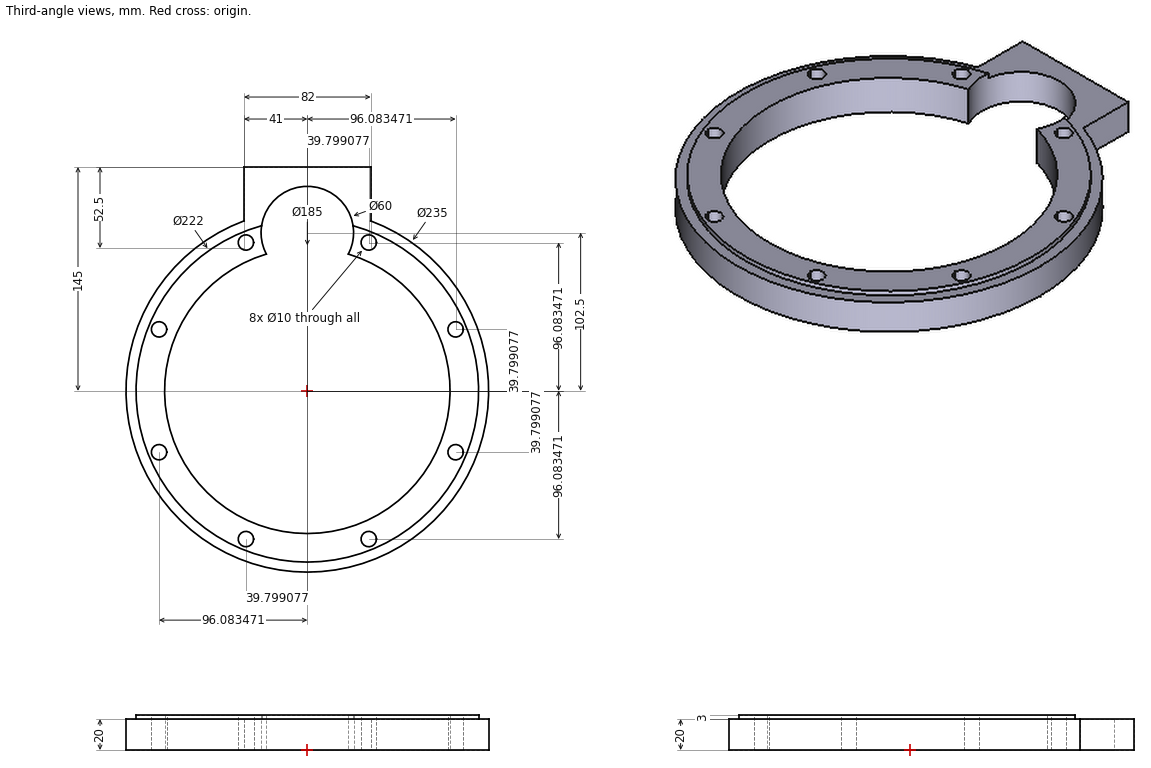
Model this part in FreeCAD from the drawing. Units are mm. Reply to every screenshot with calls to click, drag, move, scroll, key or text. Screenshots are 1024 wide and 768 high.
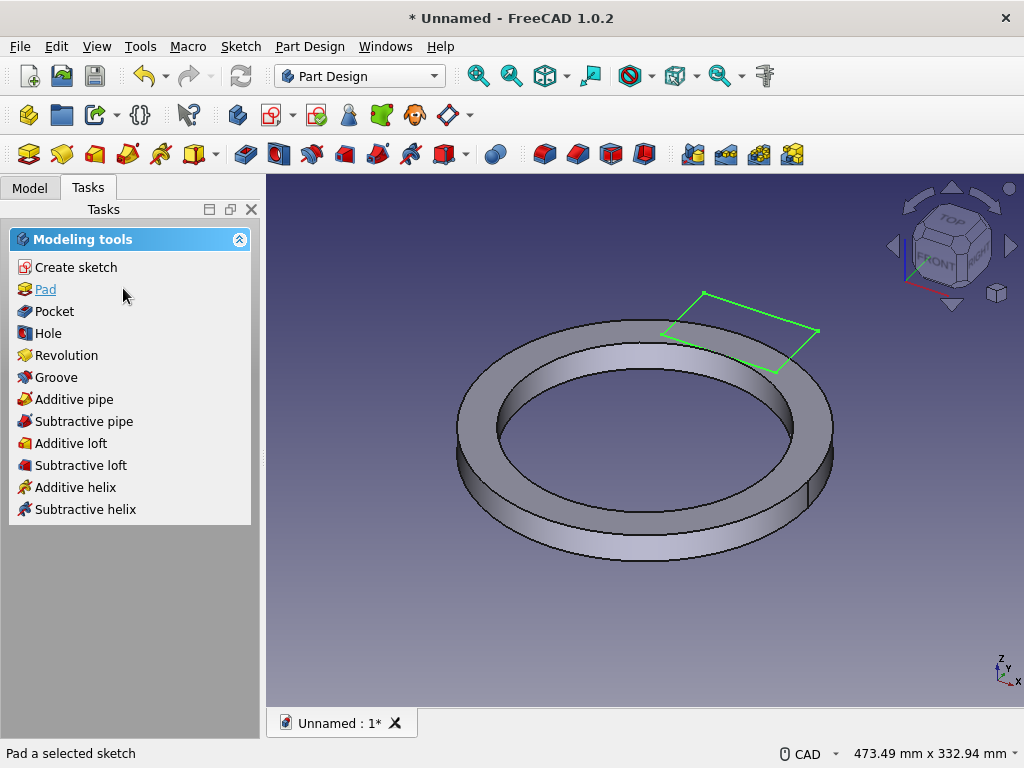
click(29, 154)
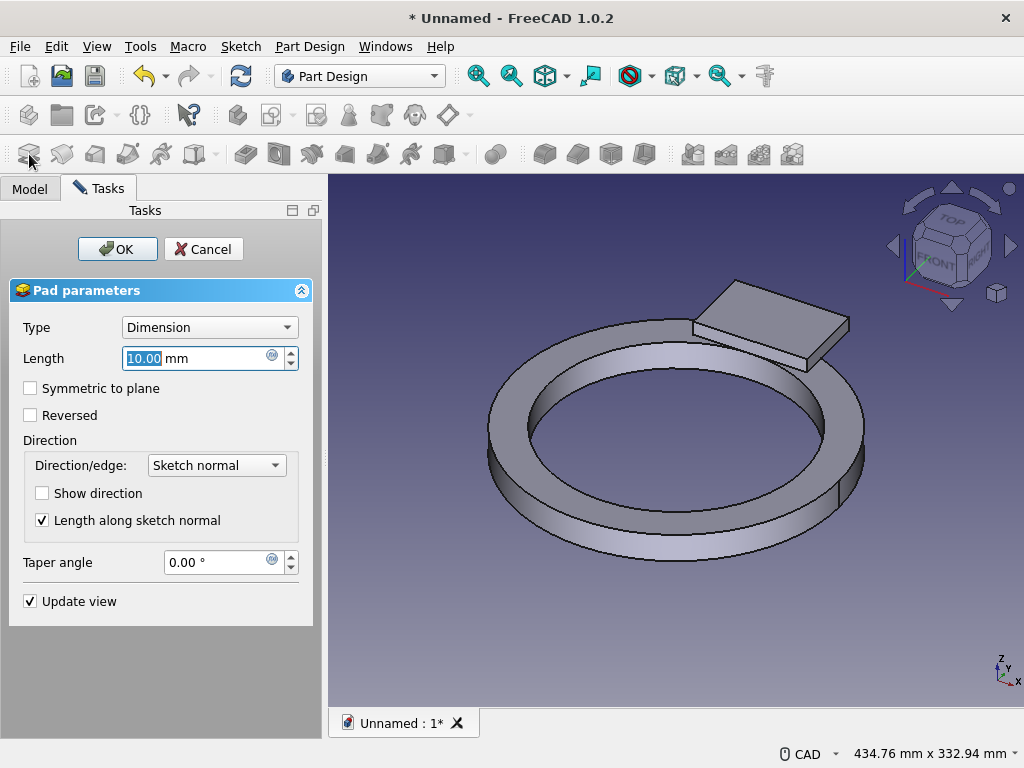
text(20)
key(Tab)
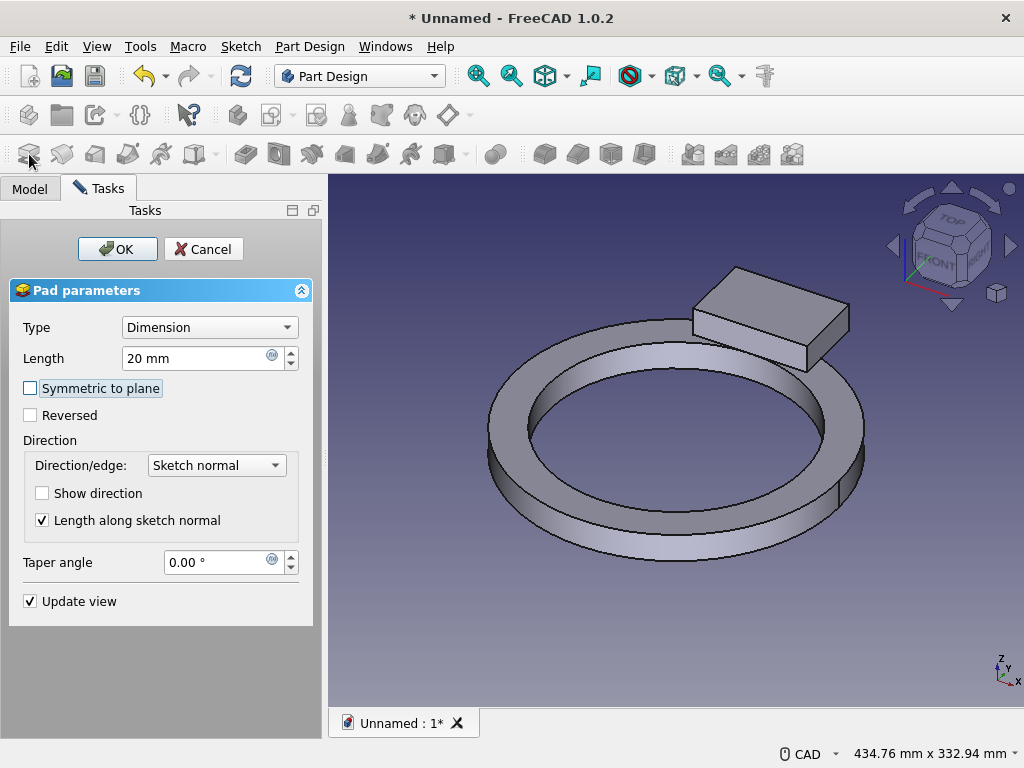
click(31, 415)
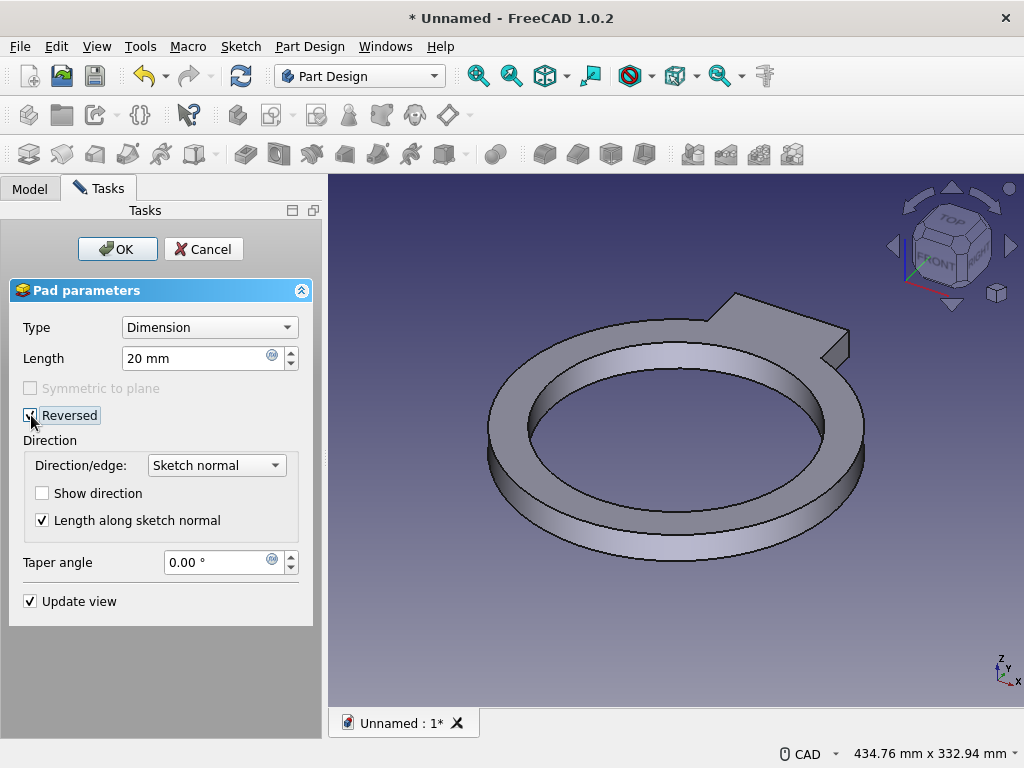
click(118, 249)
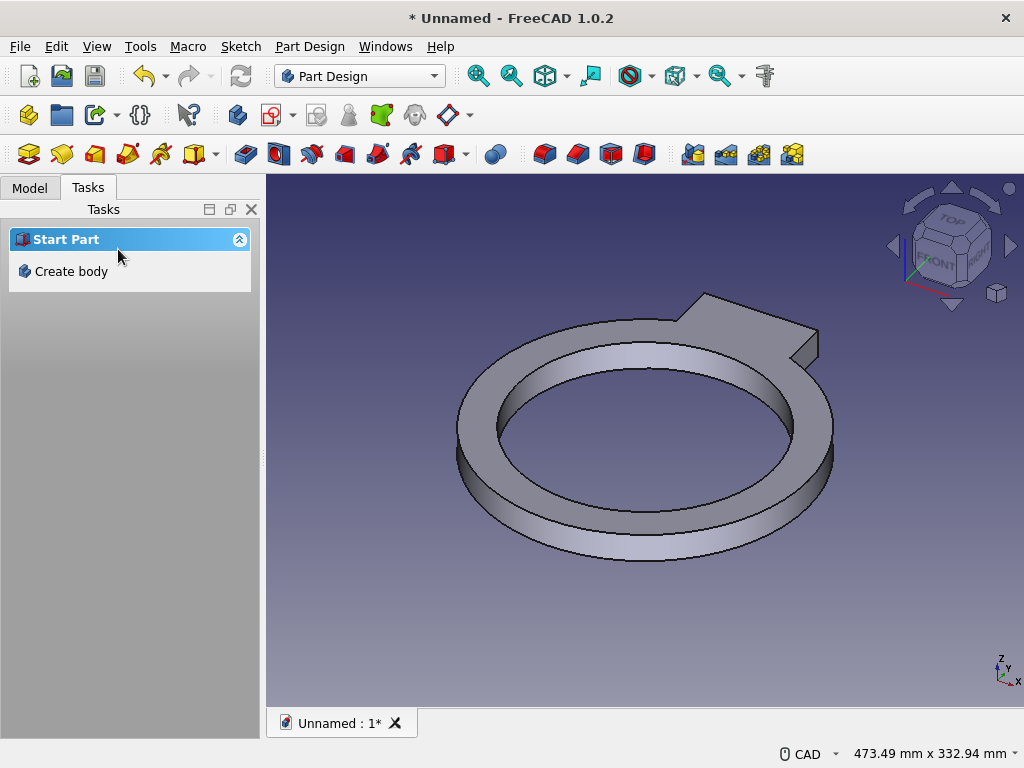
click(746, 326)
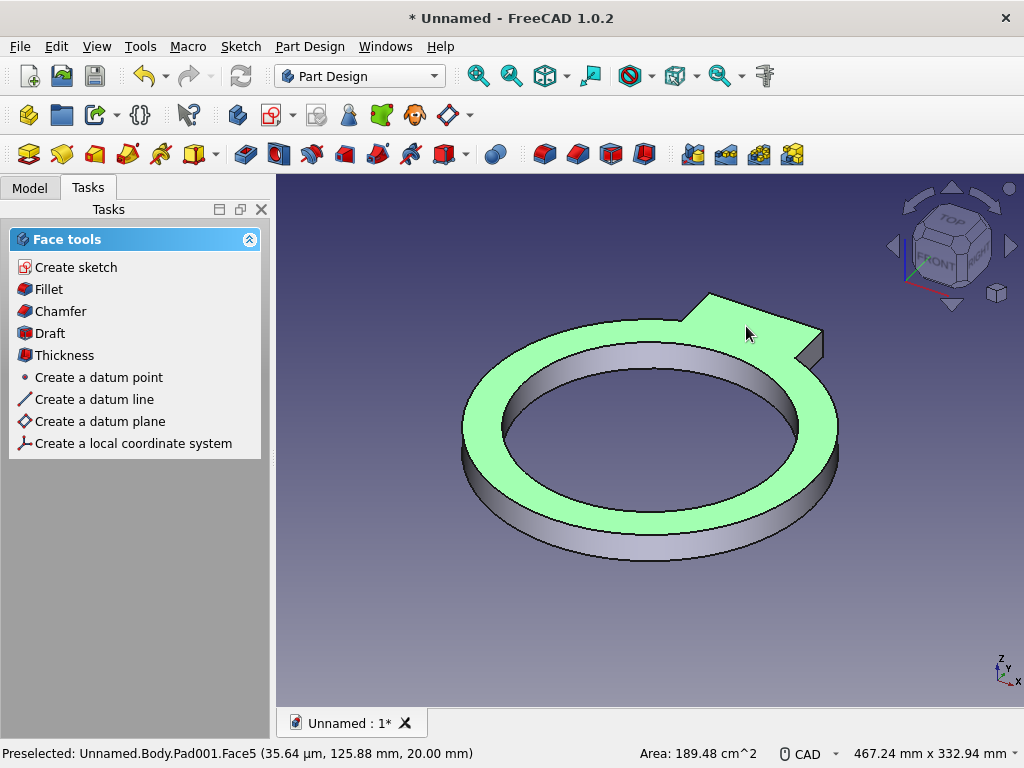
click(270, 116)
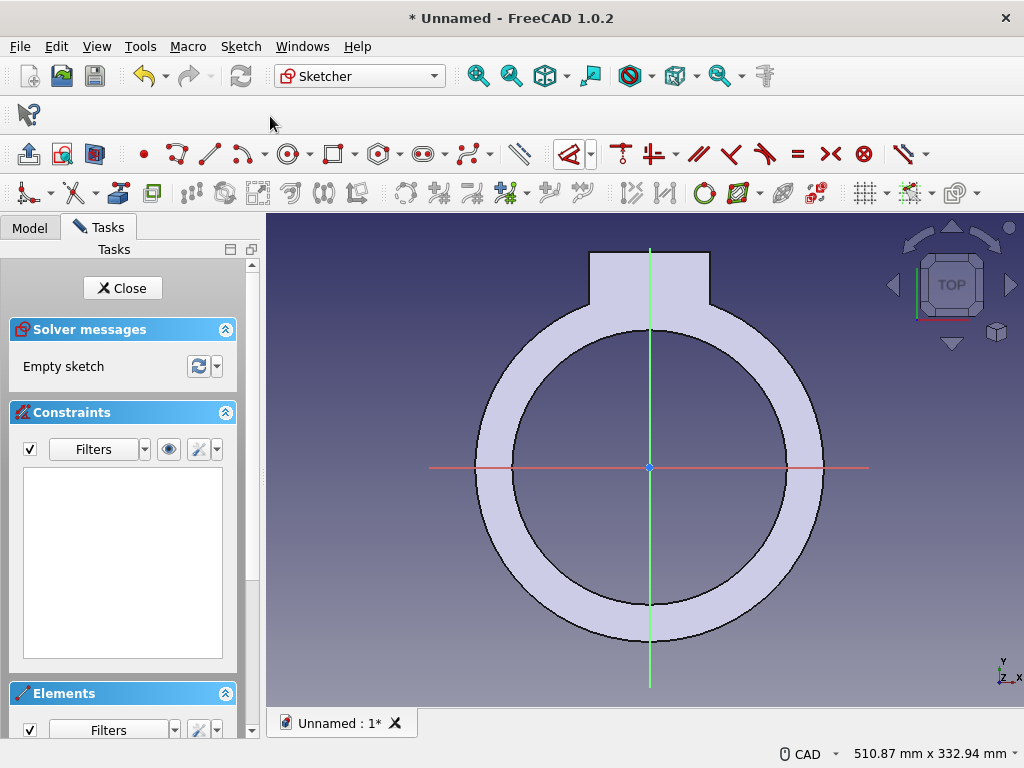
click(288, 154)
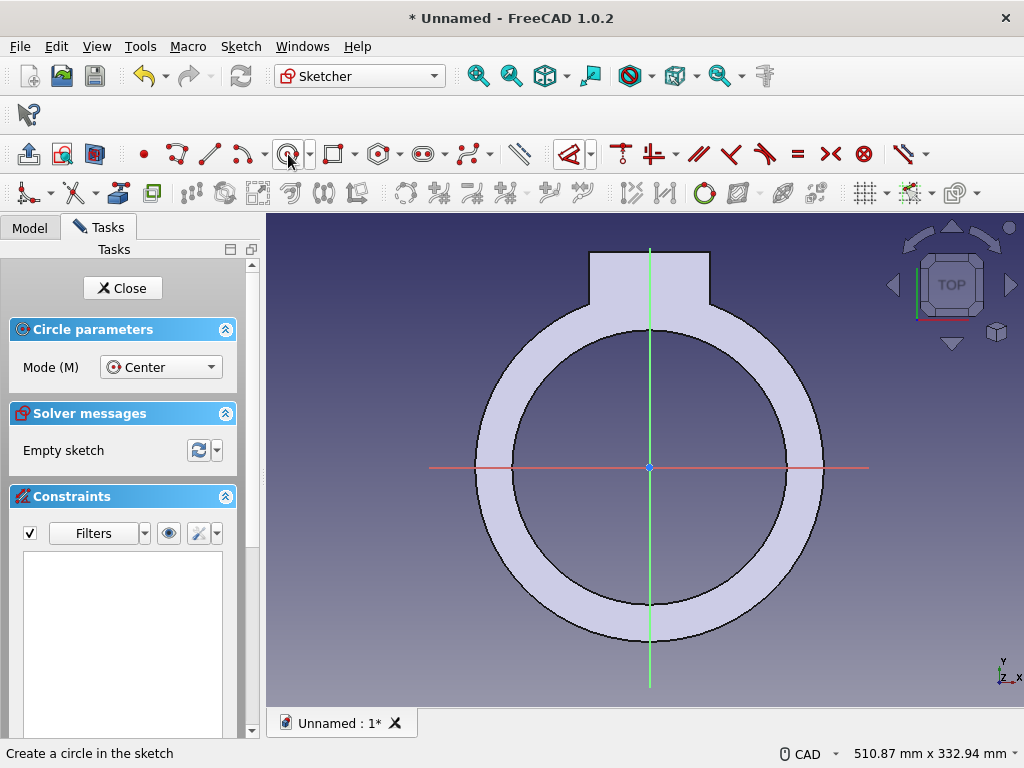
click(650, 468)
click(766, 351)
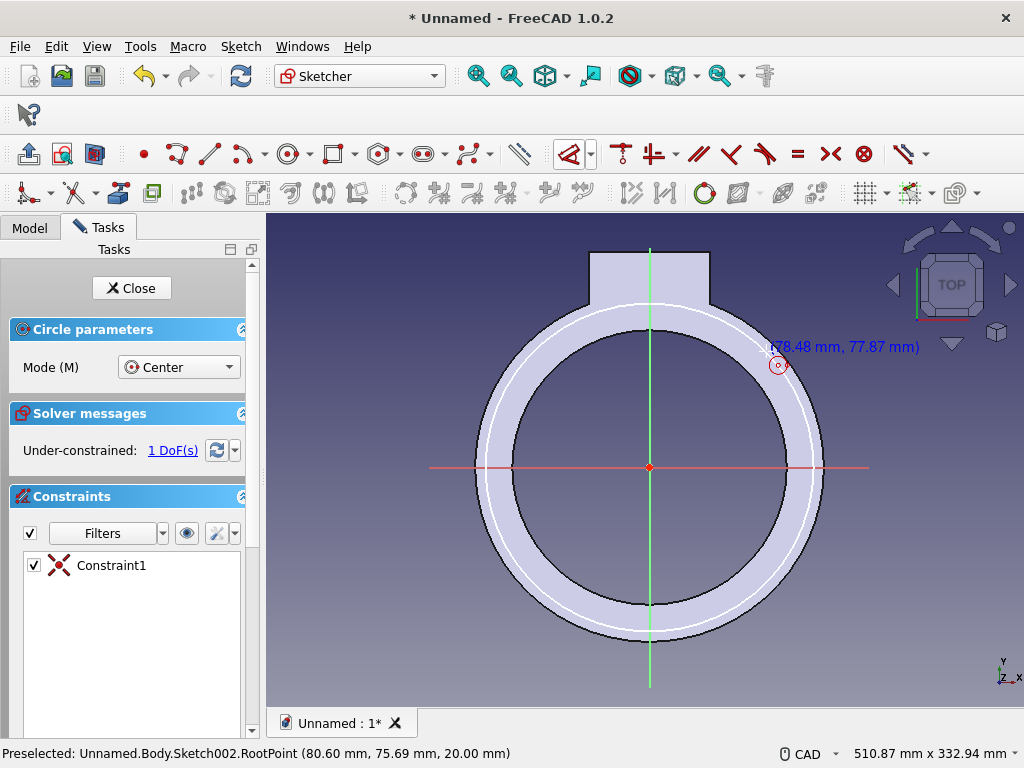
click(650, 468)
click(747, 370)
key(Escape)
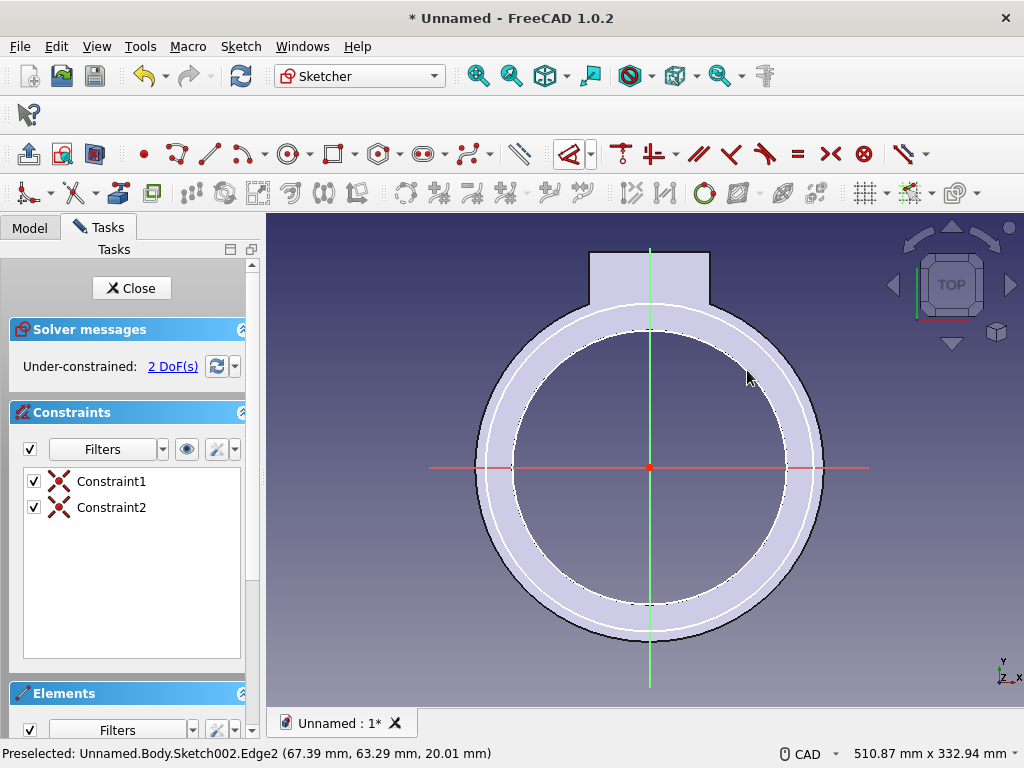
click(765, 351)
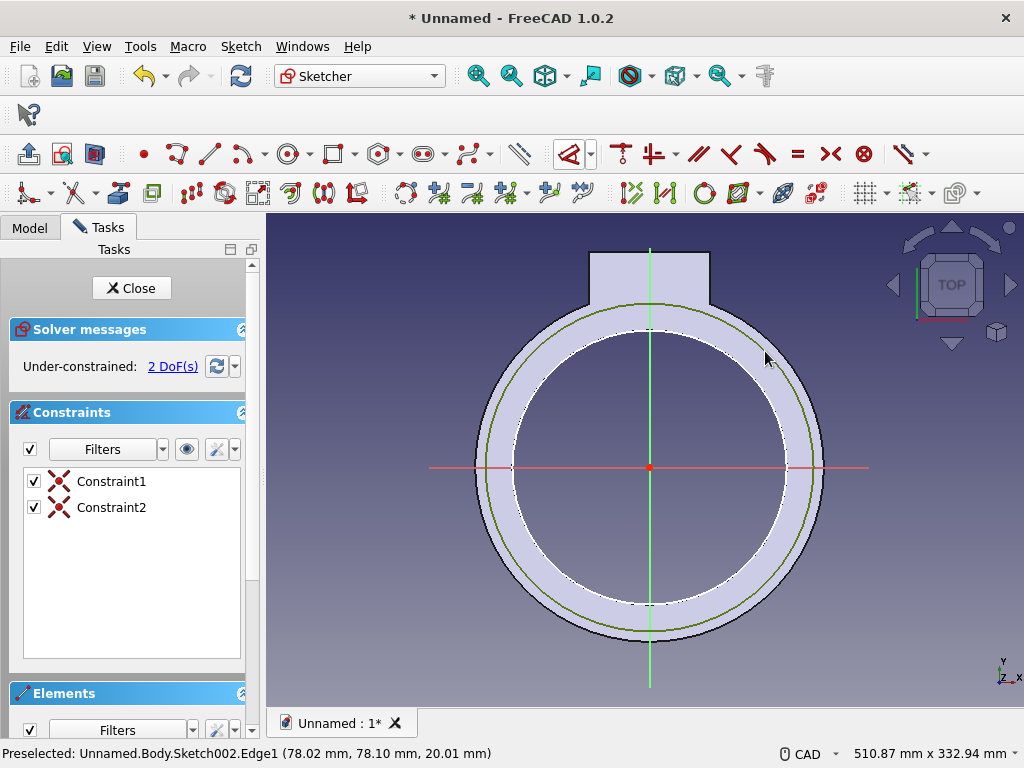
key(k)
key(o)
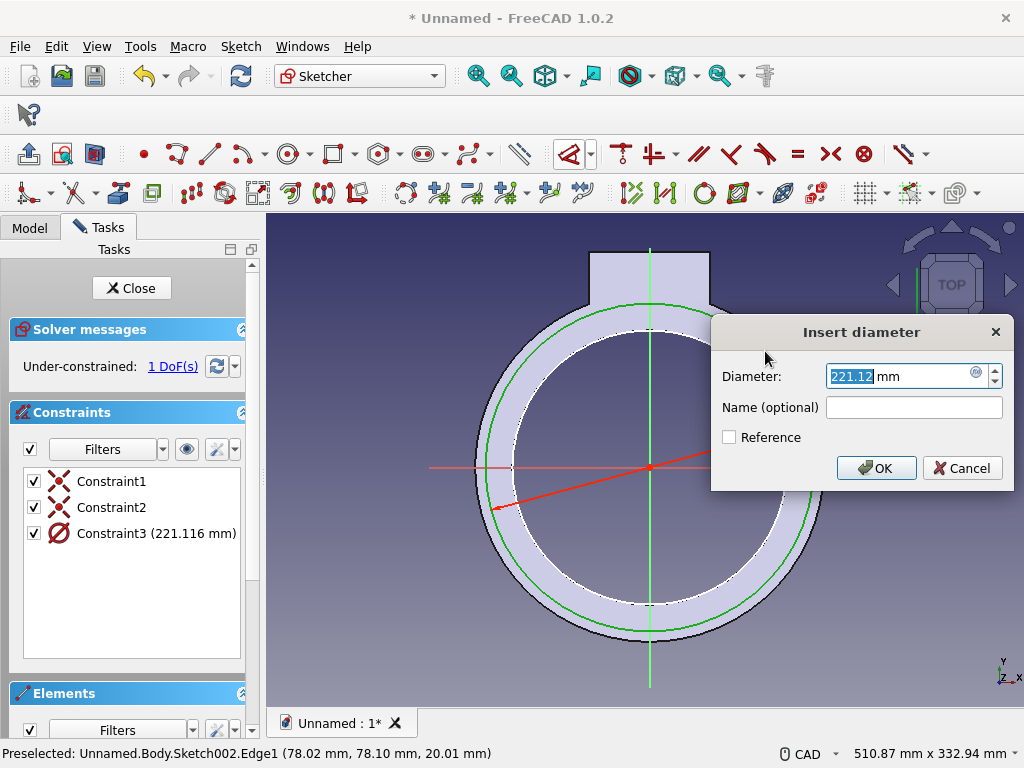
text(222)
key(Return)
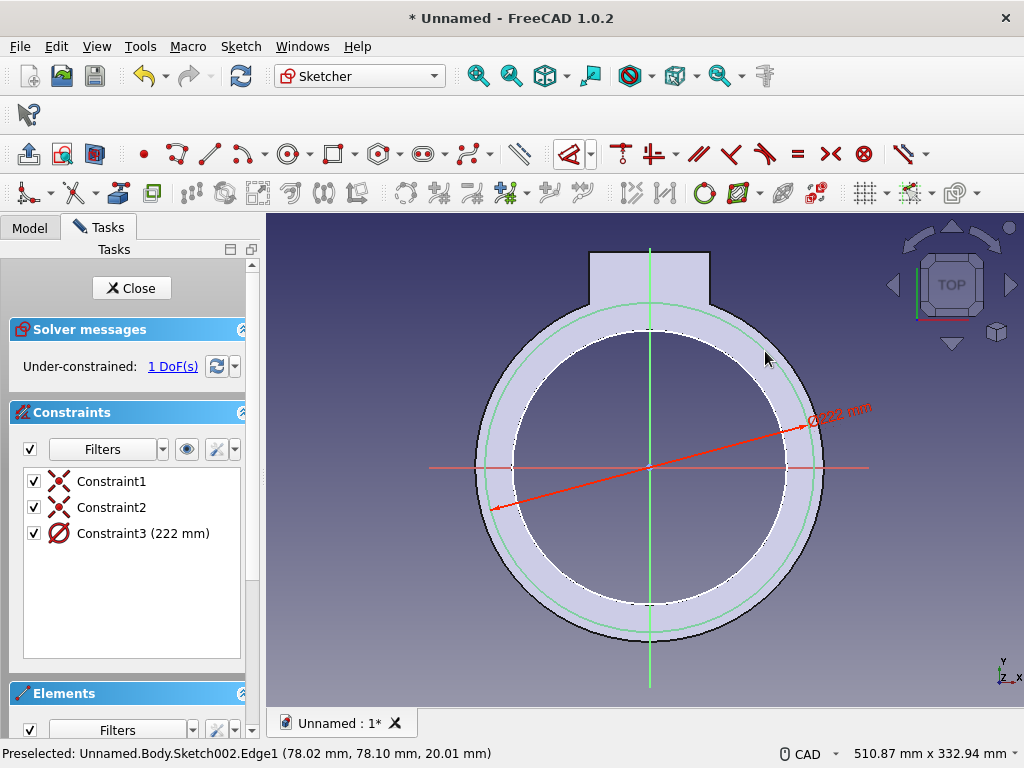
click(746, 370)